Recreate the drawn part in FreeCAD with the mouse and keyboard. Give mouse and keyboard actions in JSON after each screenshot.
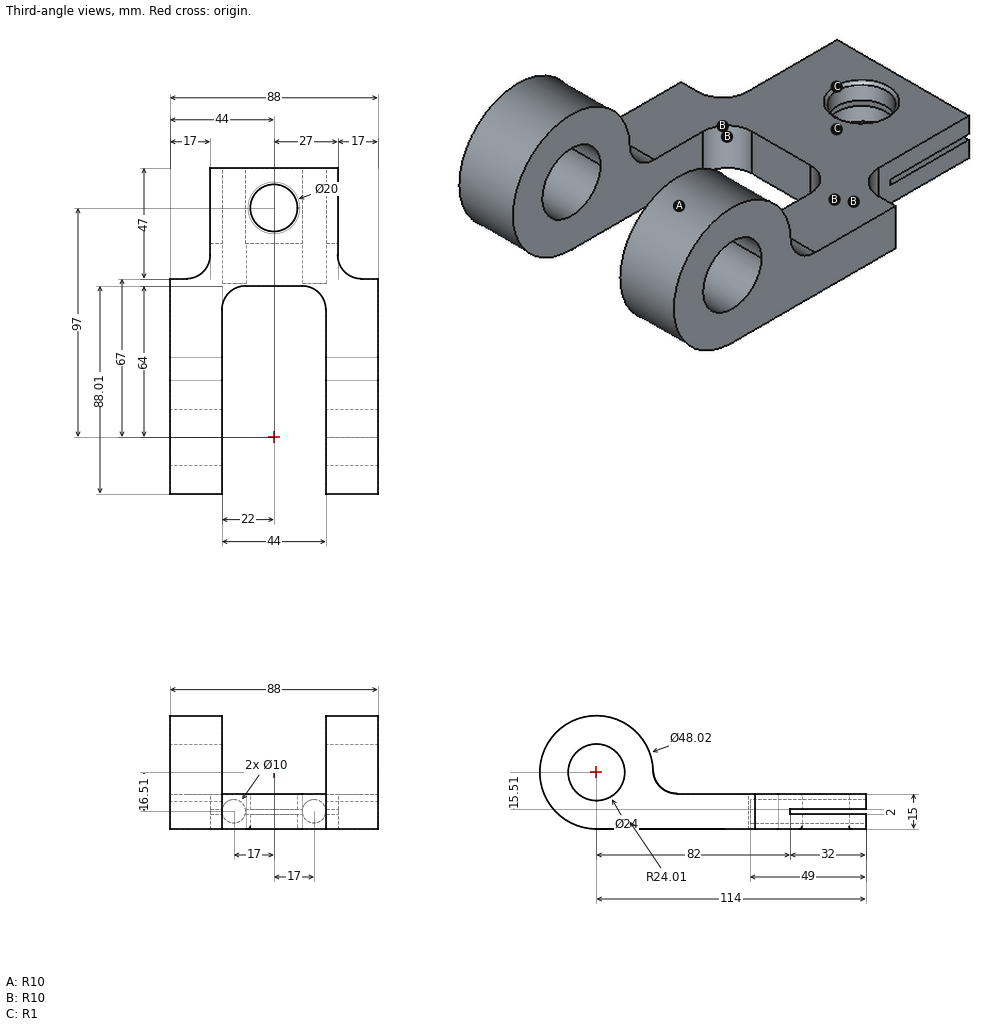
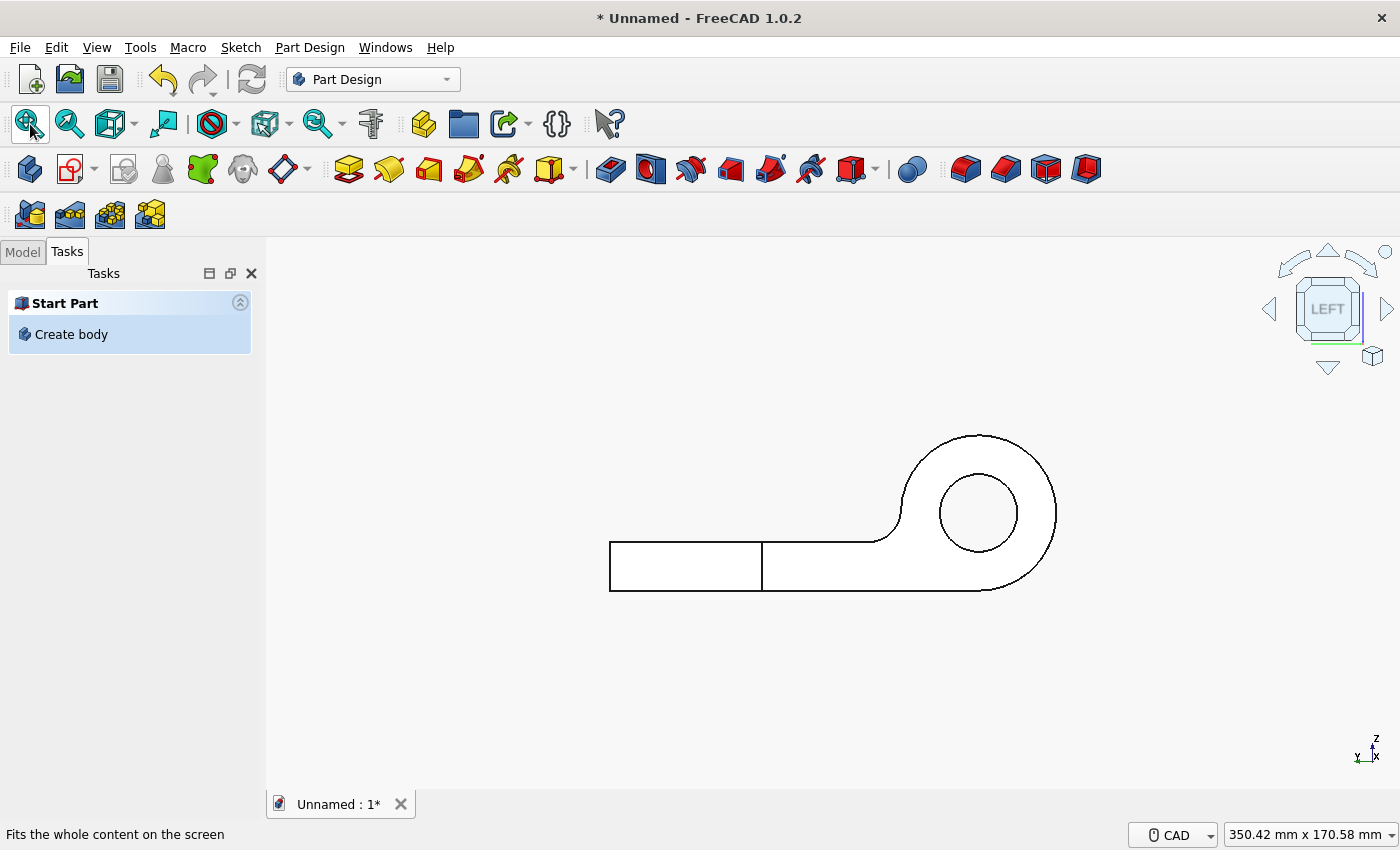
{"action": "key", "text": "v 3"}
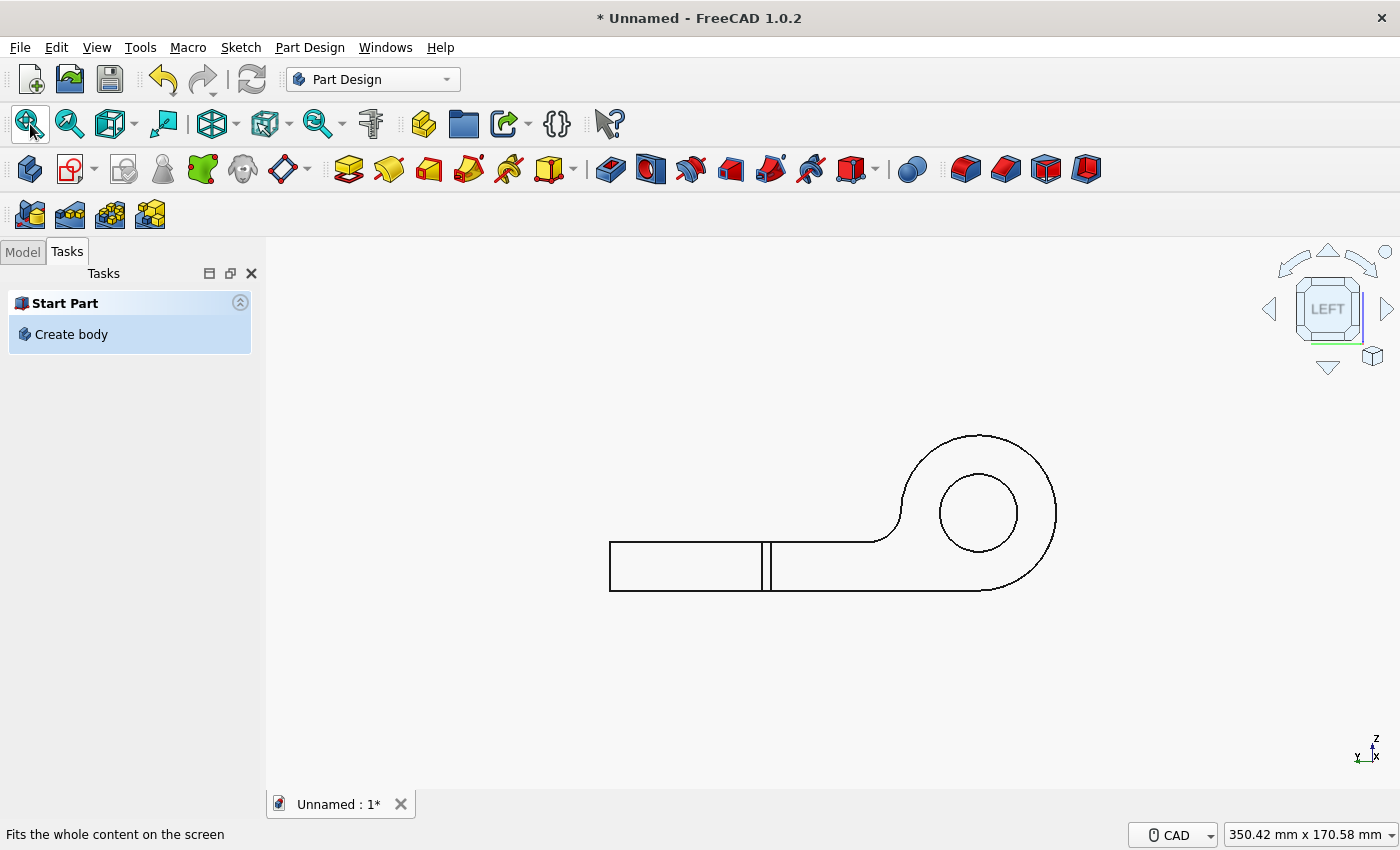
{"action": "key", "text": "0"}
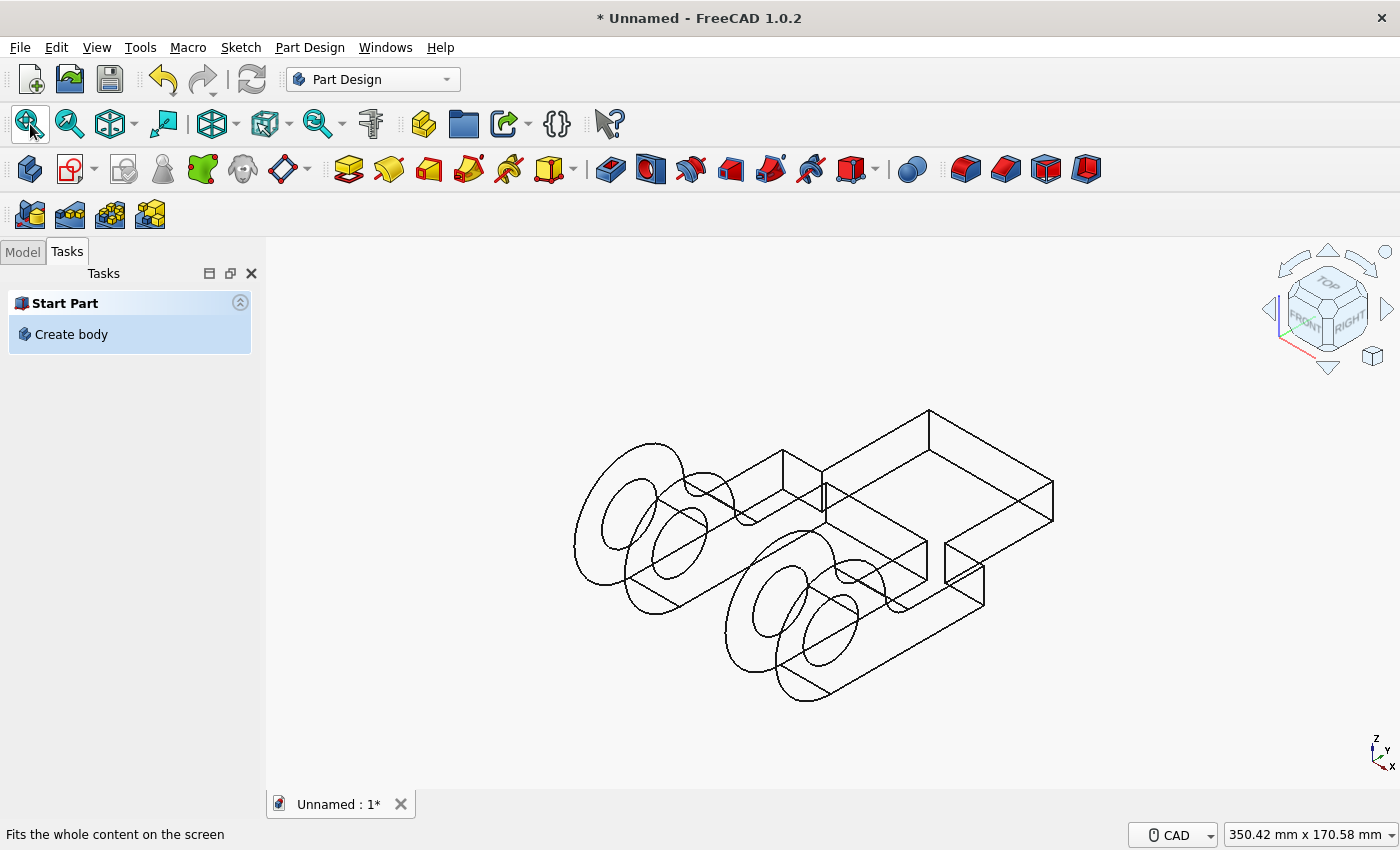
{"action": "left_click", "coordinate": [826, 501]}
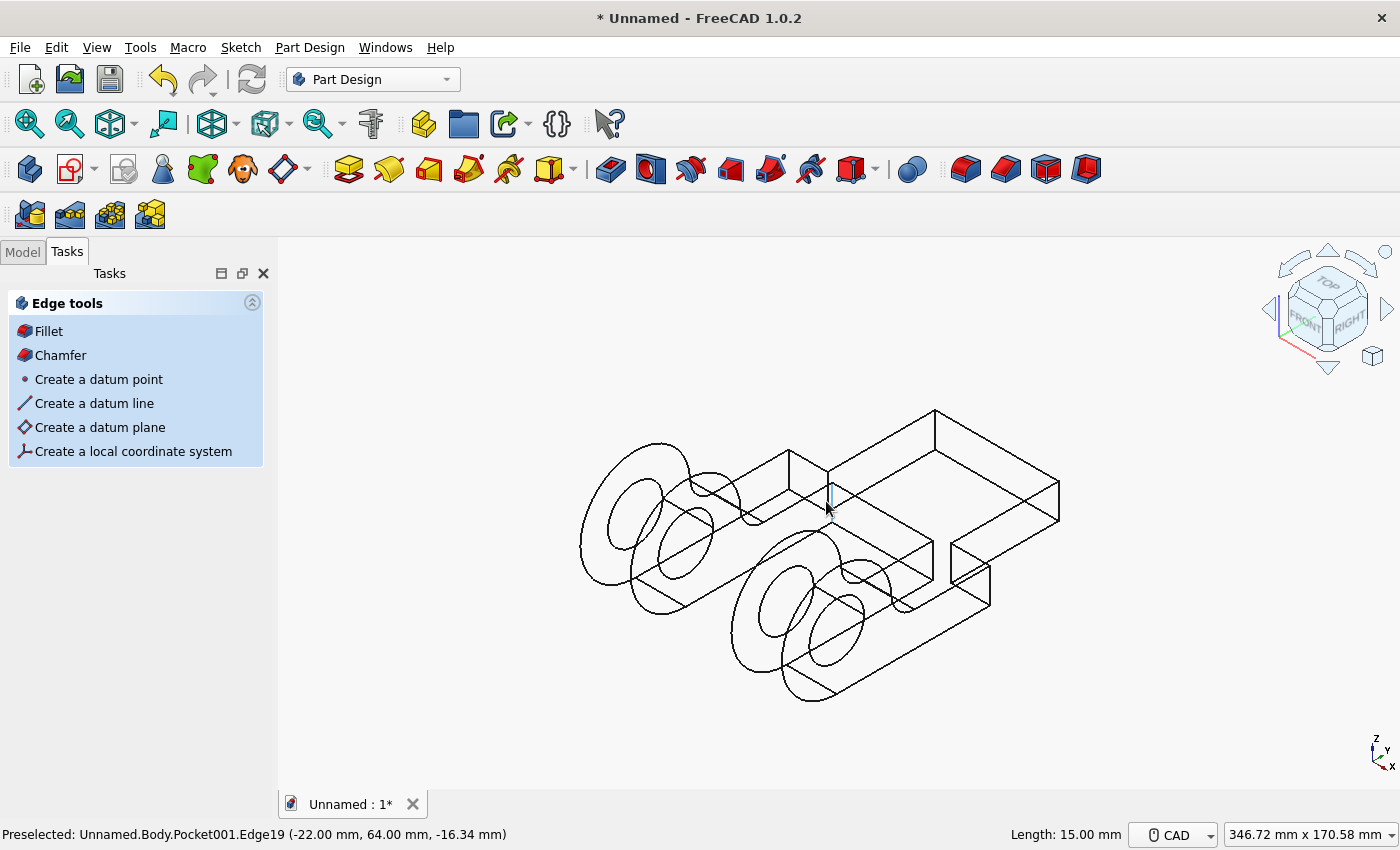
{"action": "left_click", "coordinate": [933, 560], "text": "ctrl"}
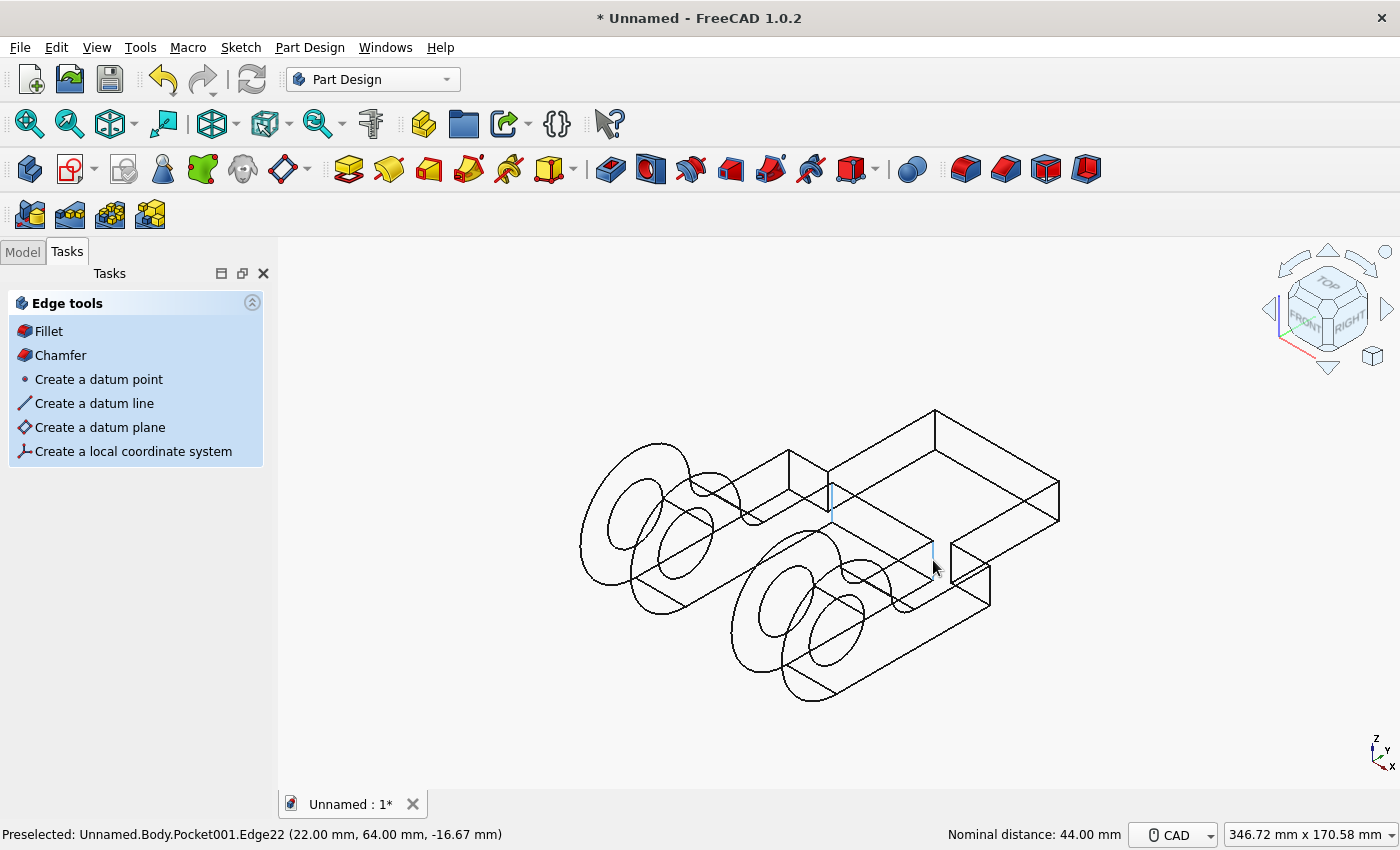
{"action": "left_click", "coordinate": [951, 562], "text": "ctrl"}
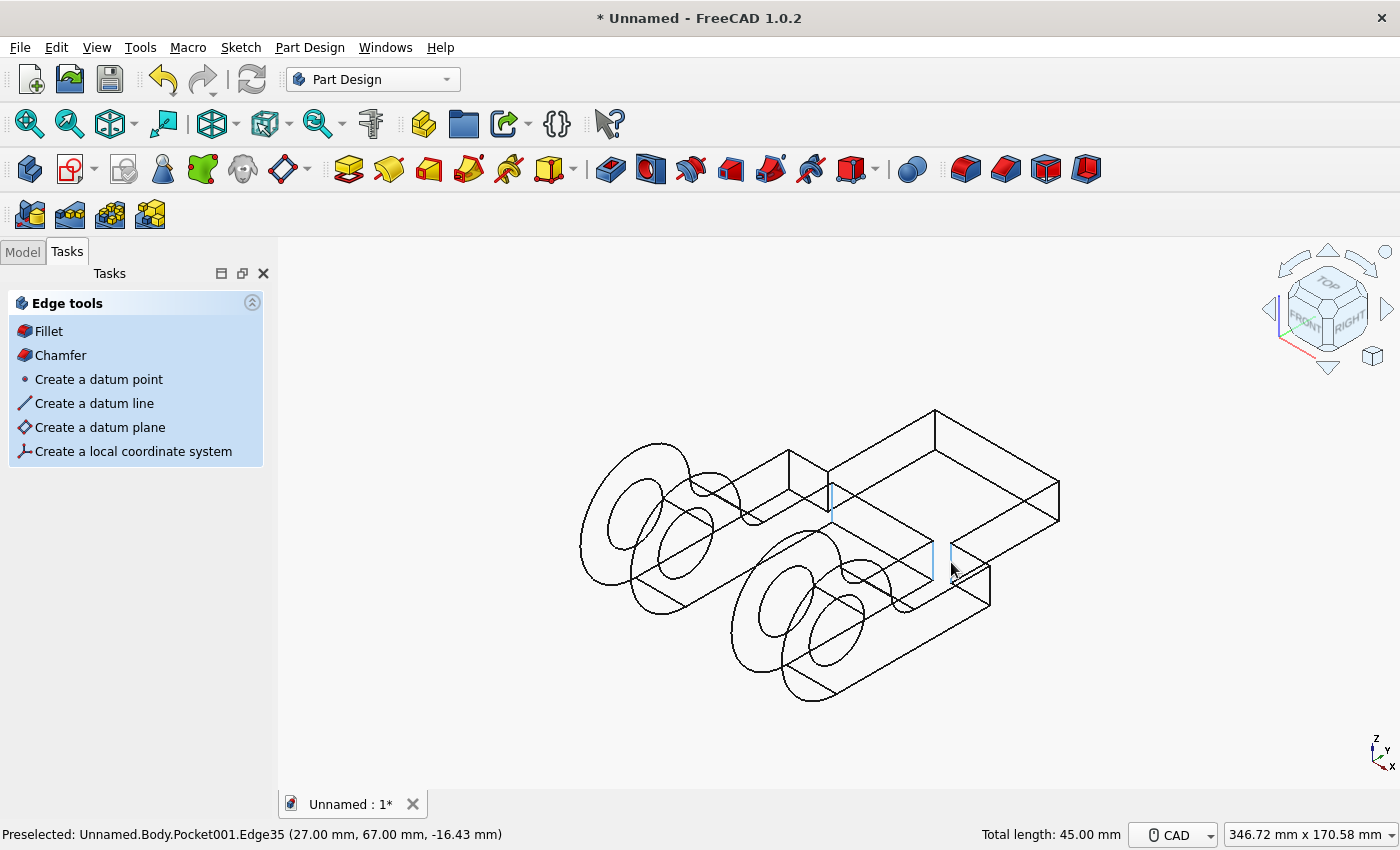
{"action": "key", "text": "2"}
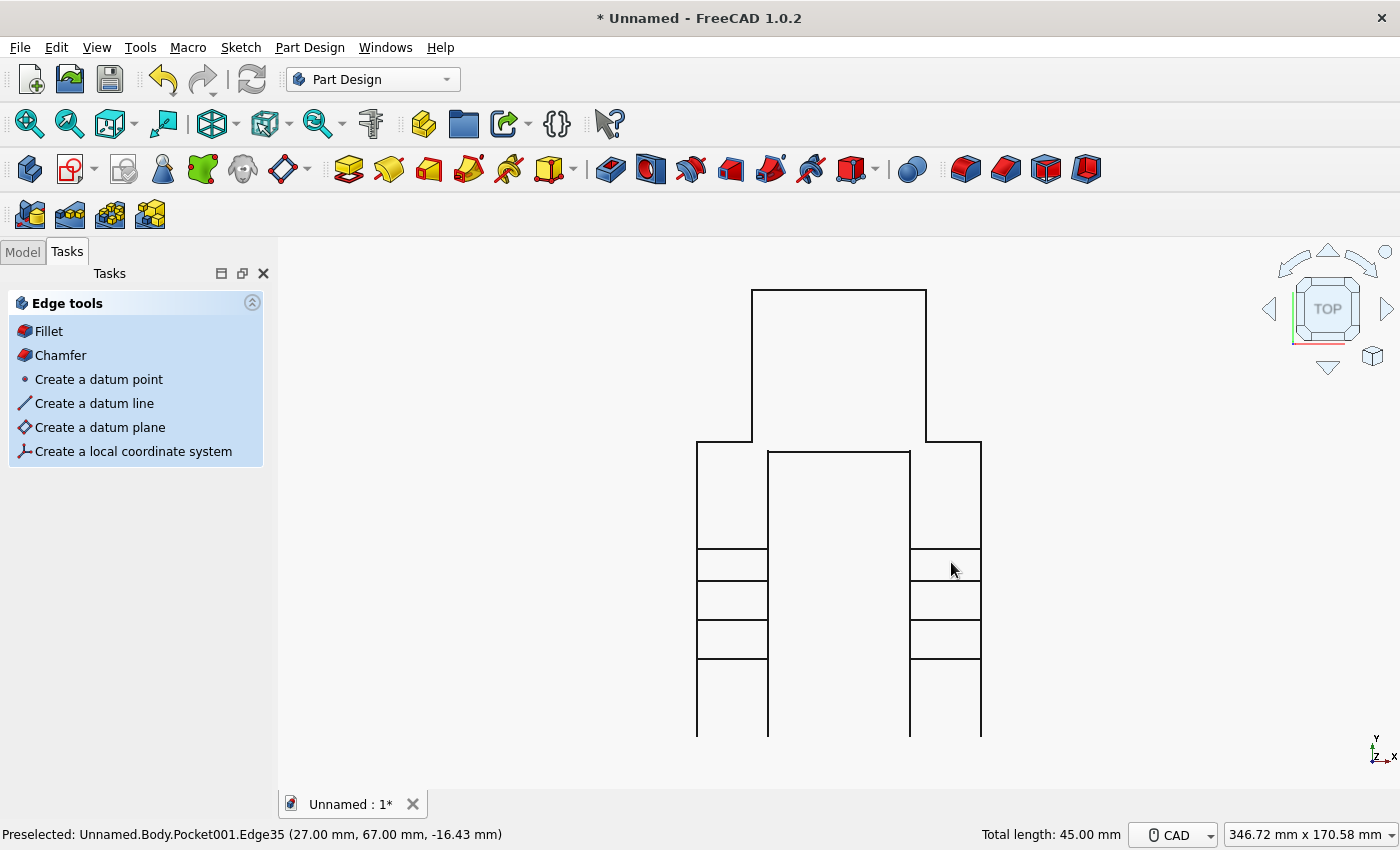
{"action": "key", "text": "1"}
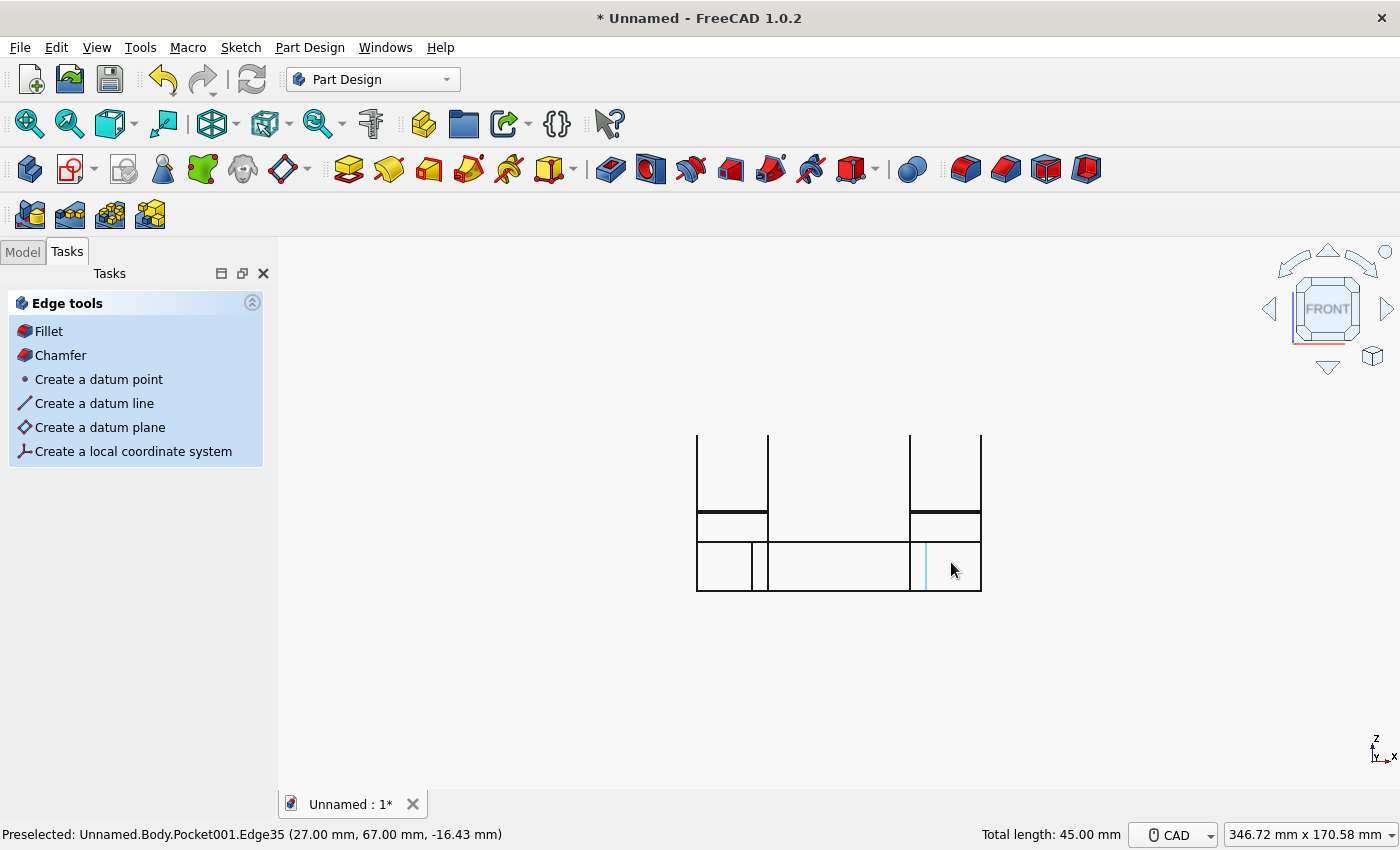
{"action": "left_click", "coordinate": [30, 124]}